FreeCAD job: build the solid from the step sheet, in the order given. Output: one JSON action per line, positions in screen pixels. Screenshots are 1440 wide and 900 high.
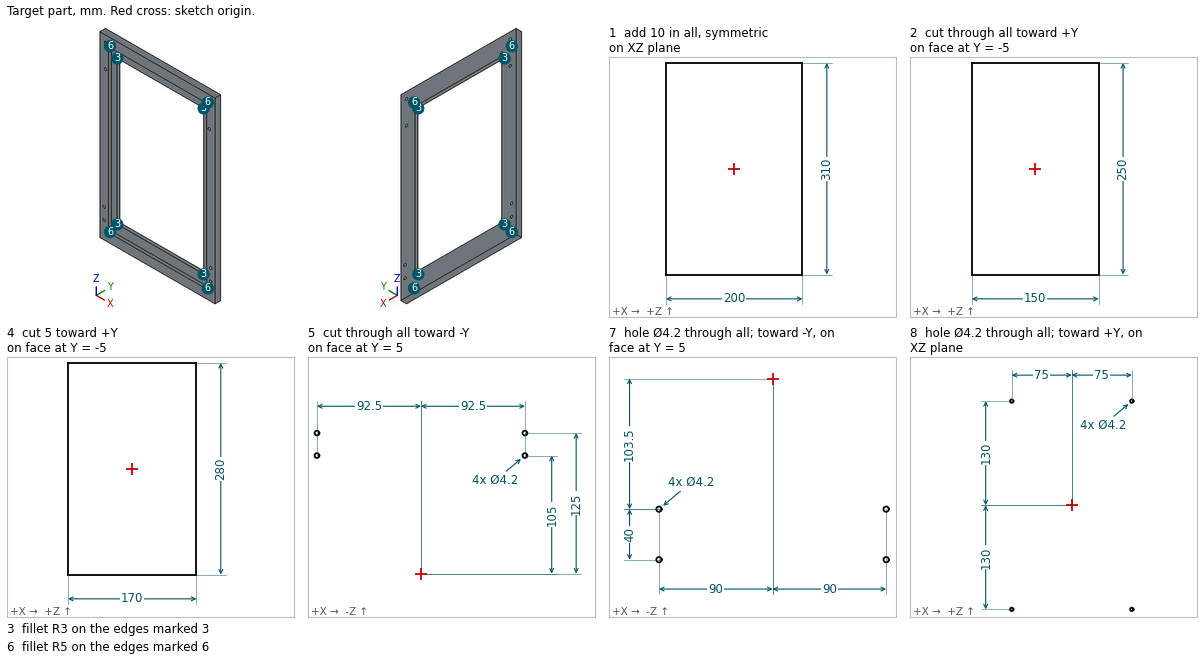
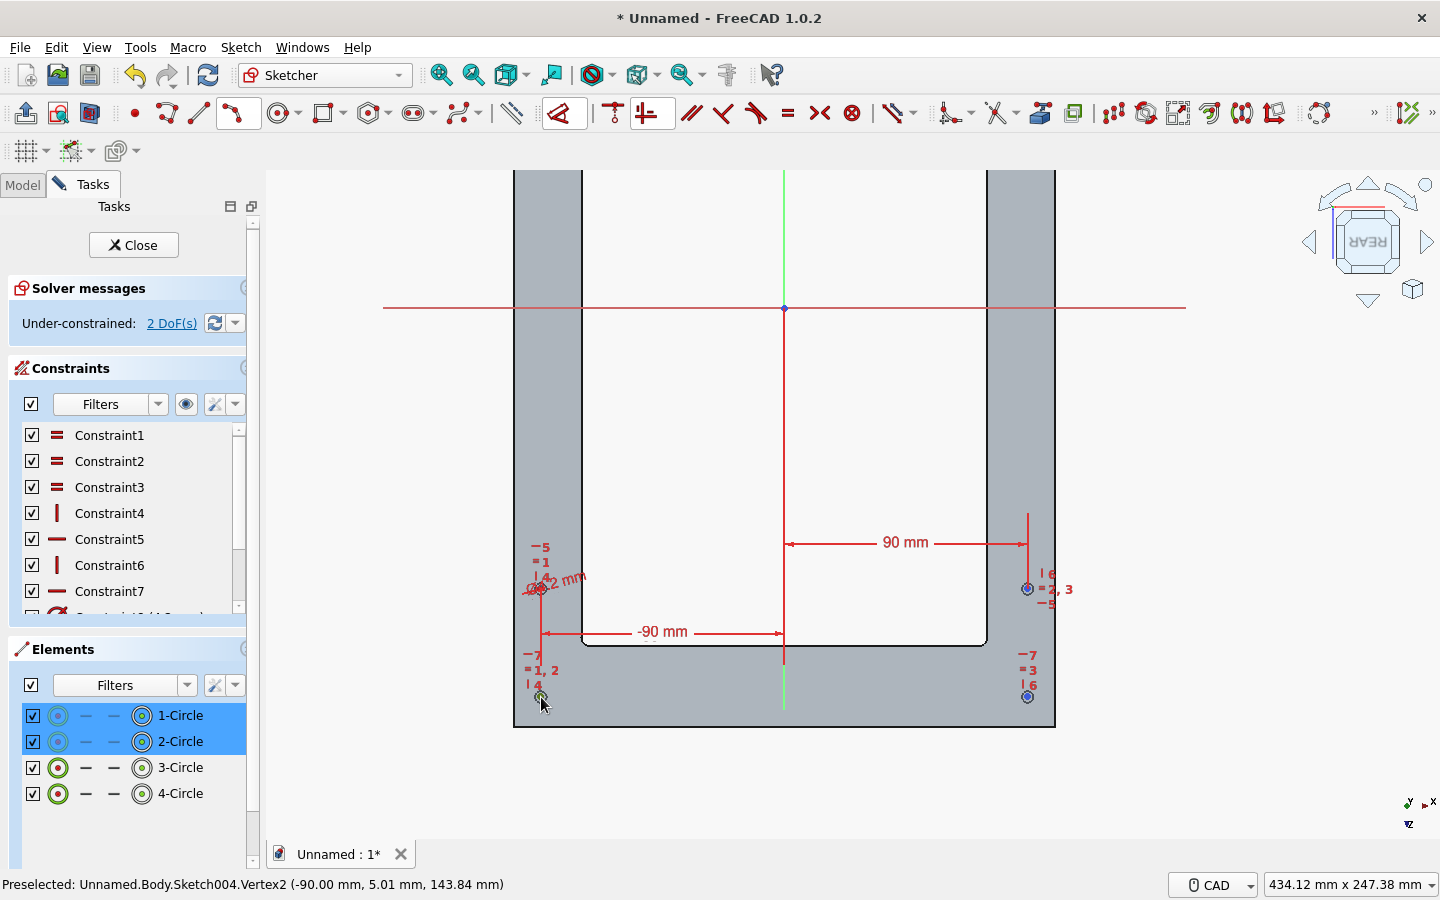
{"action": "key", "text": "i"}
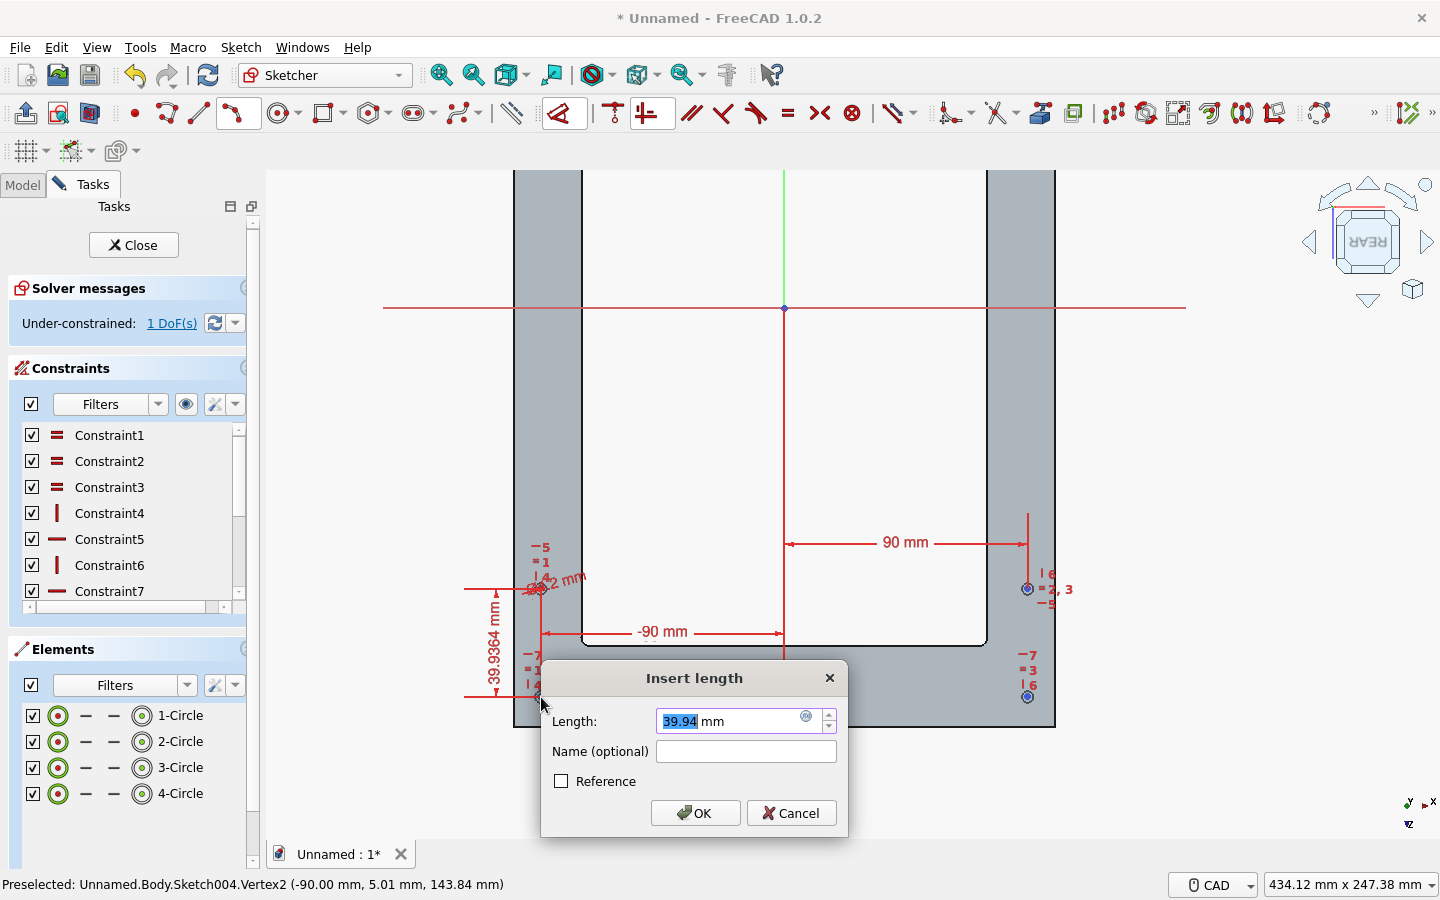
{"action": "type", "text": "40"}
{"action": "key", "text": "Return"}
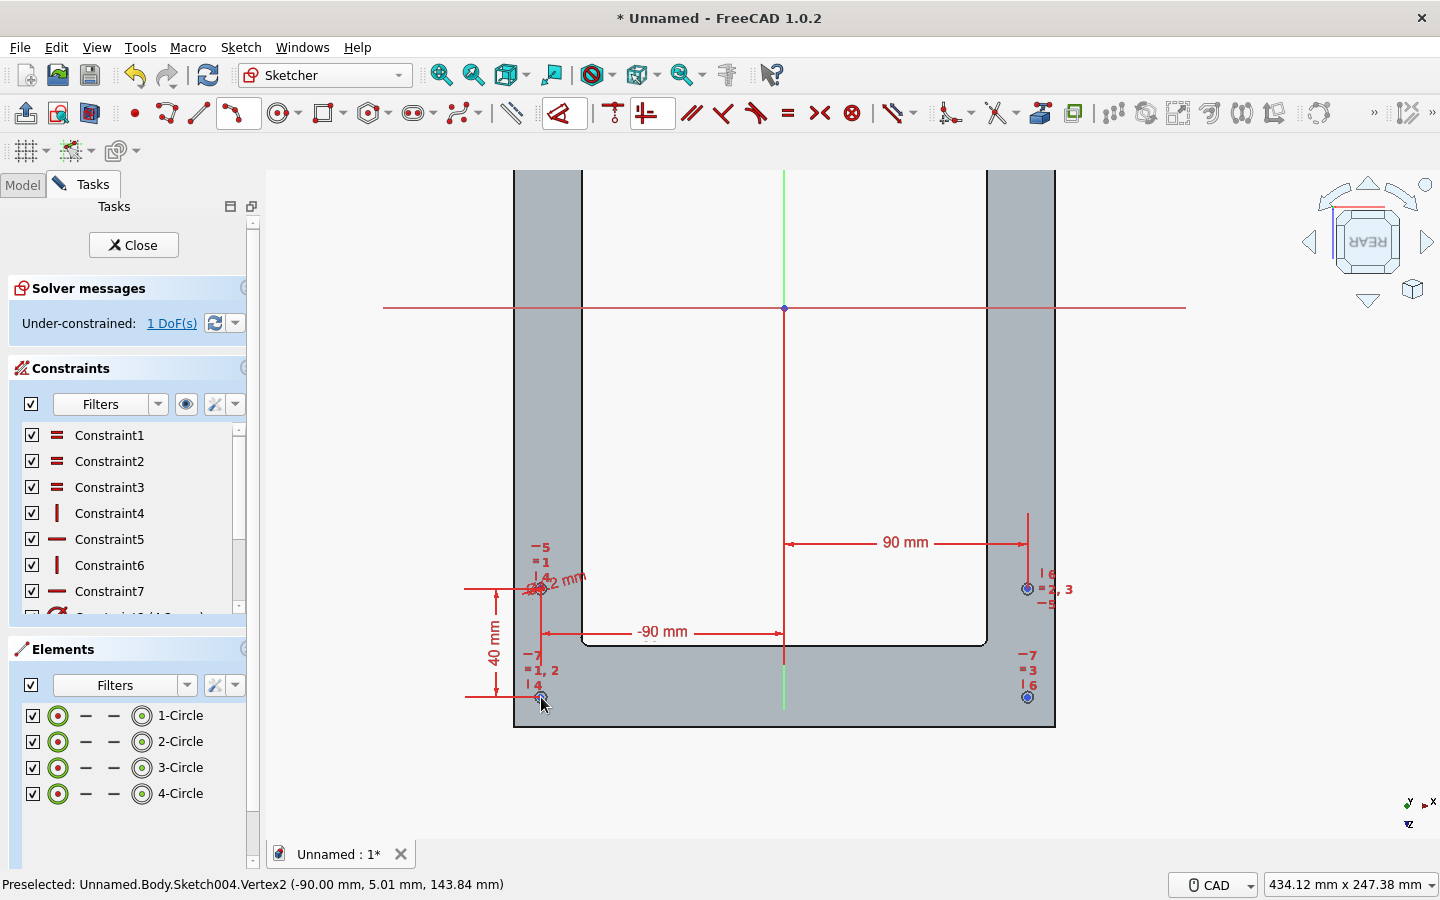
{"action": "left_click", "coordinate": [541, 589]}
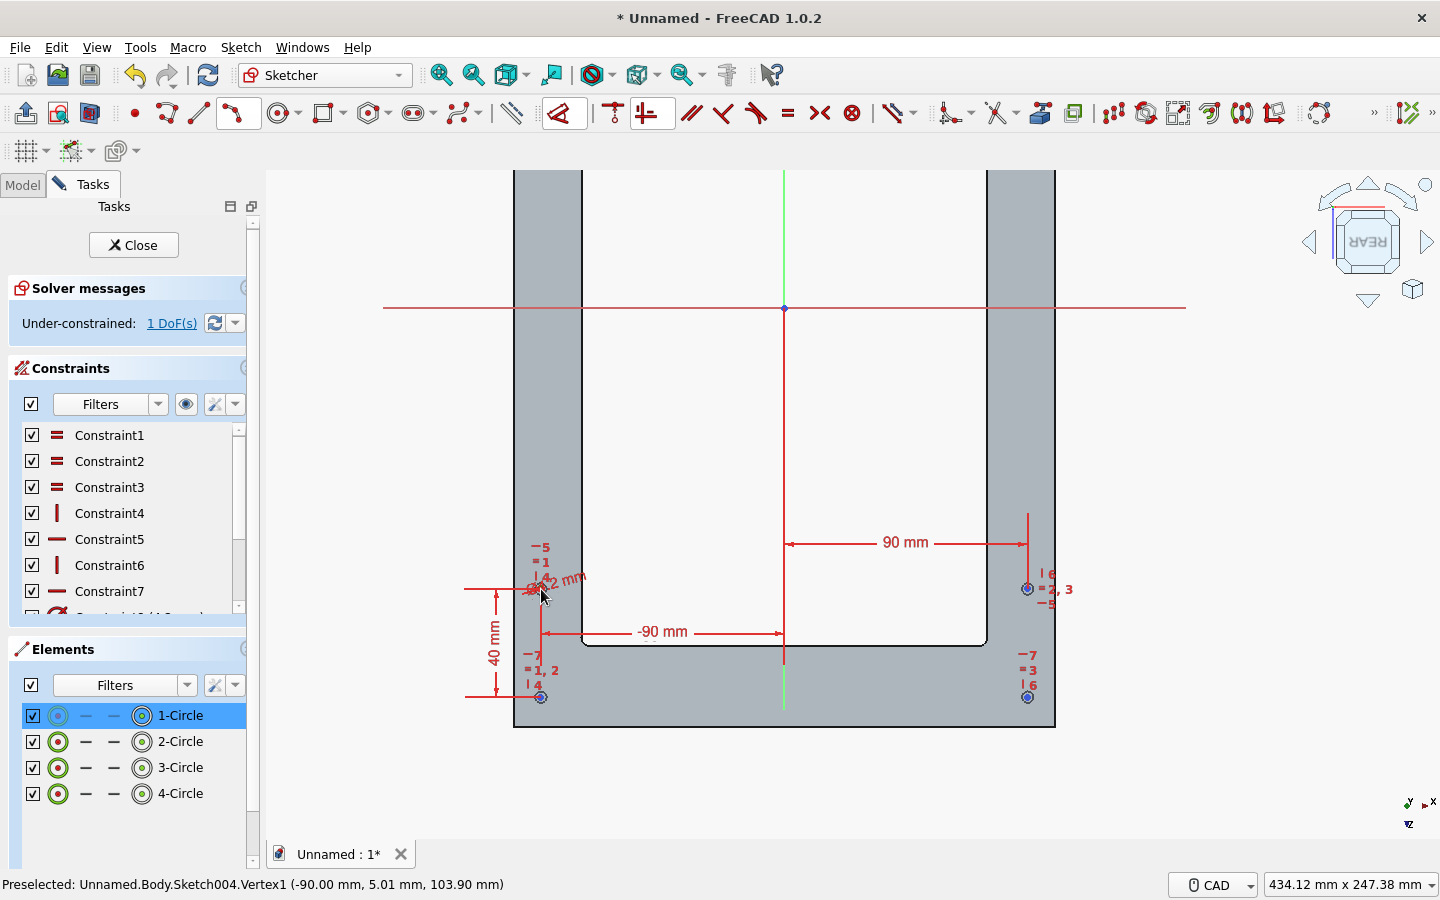
{"action": "key", "text": "i"}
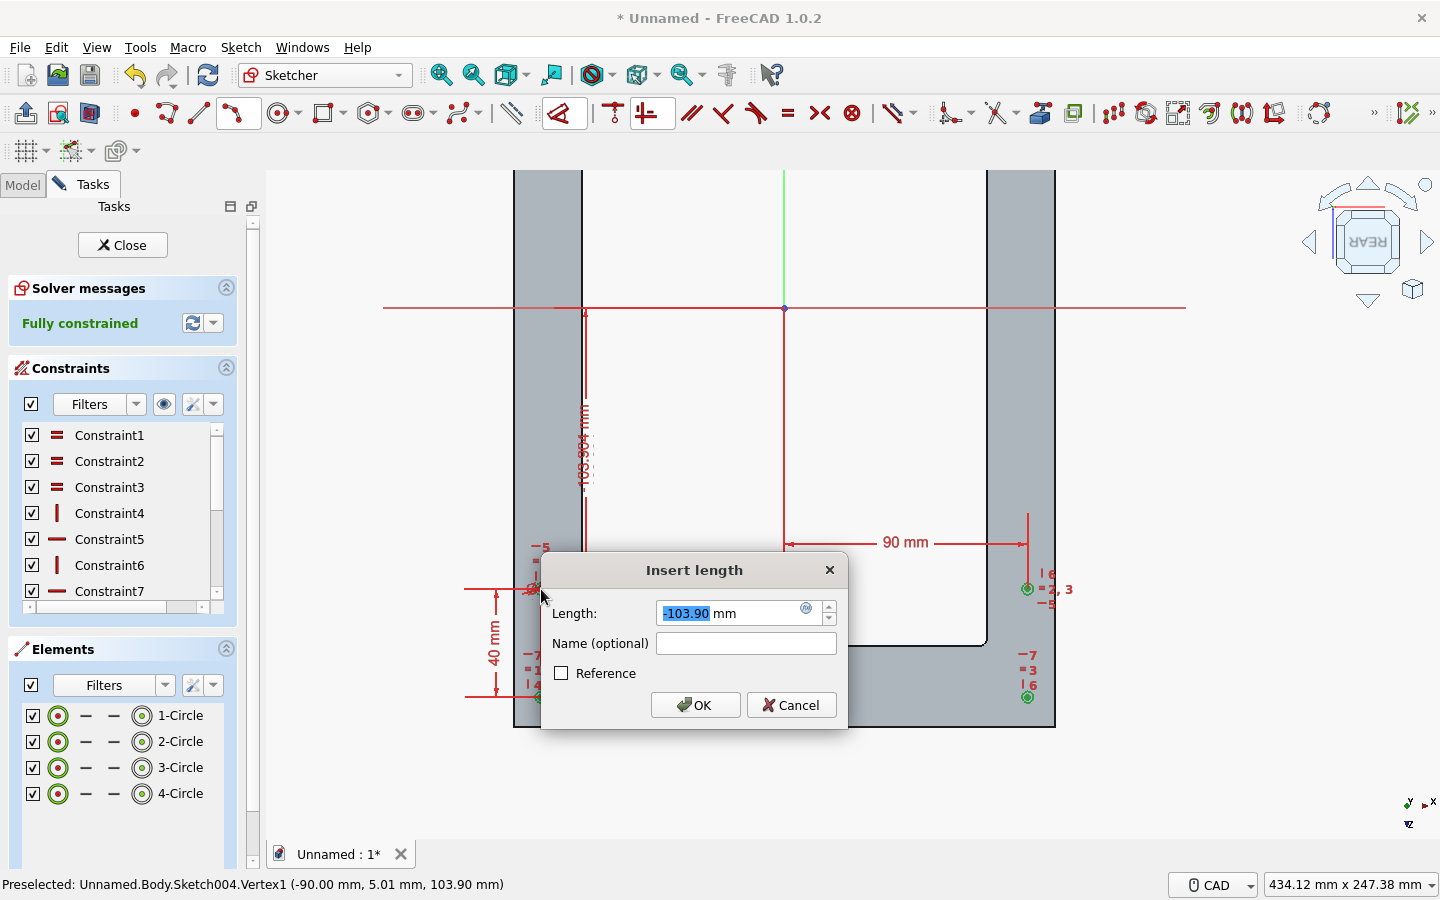
{"action": "type", "text": "-103.5"}
{"action": "key", "text": "Return"}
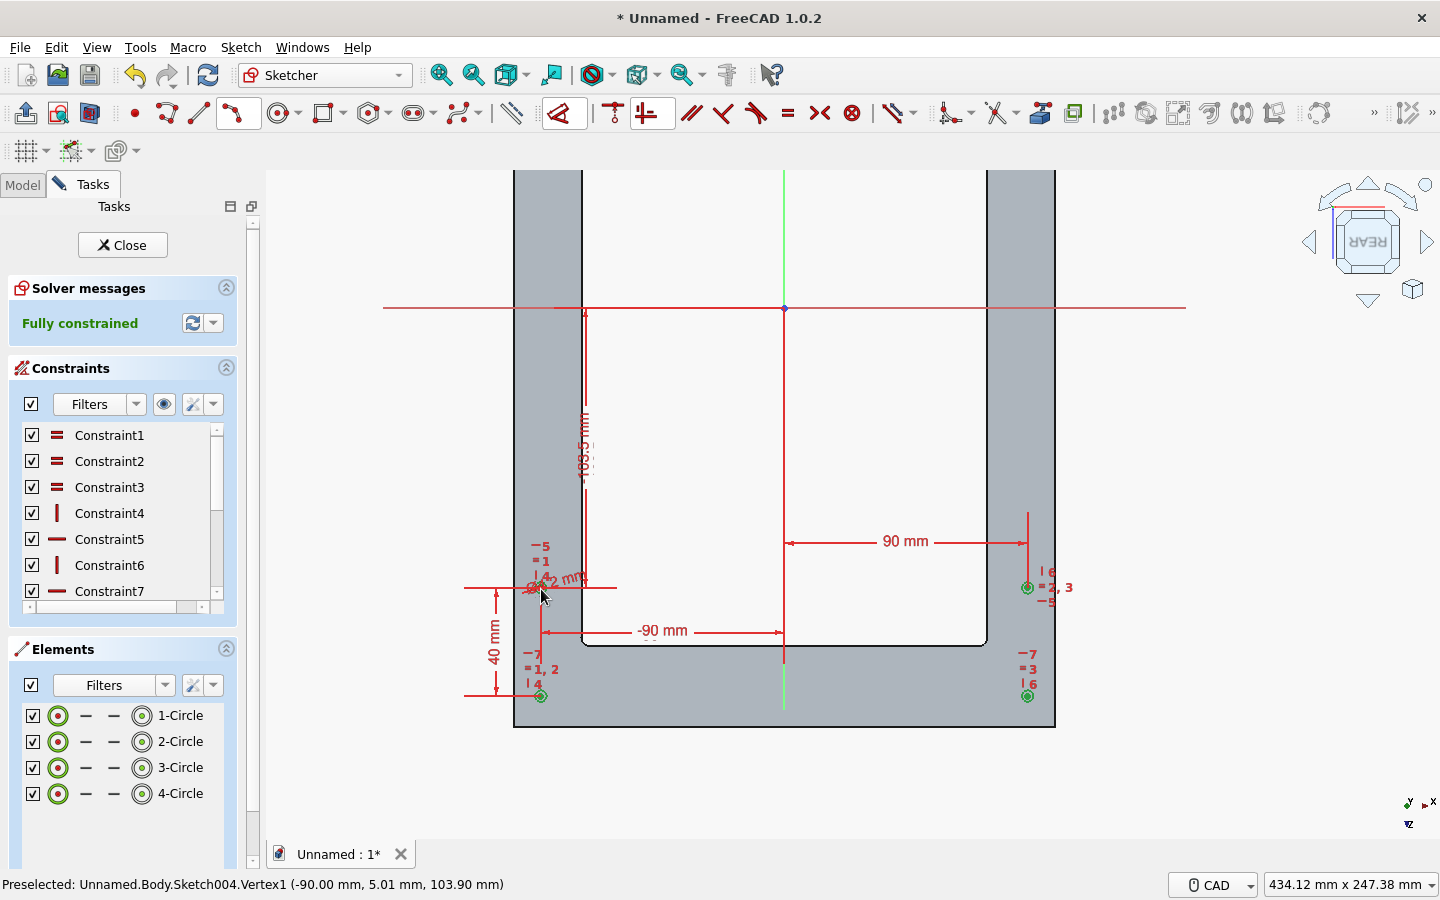
{"action": "left_click", "coordinate": [123, 245]}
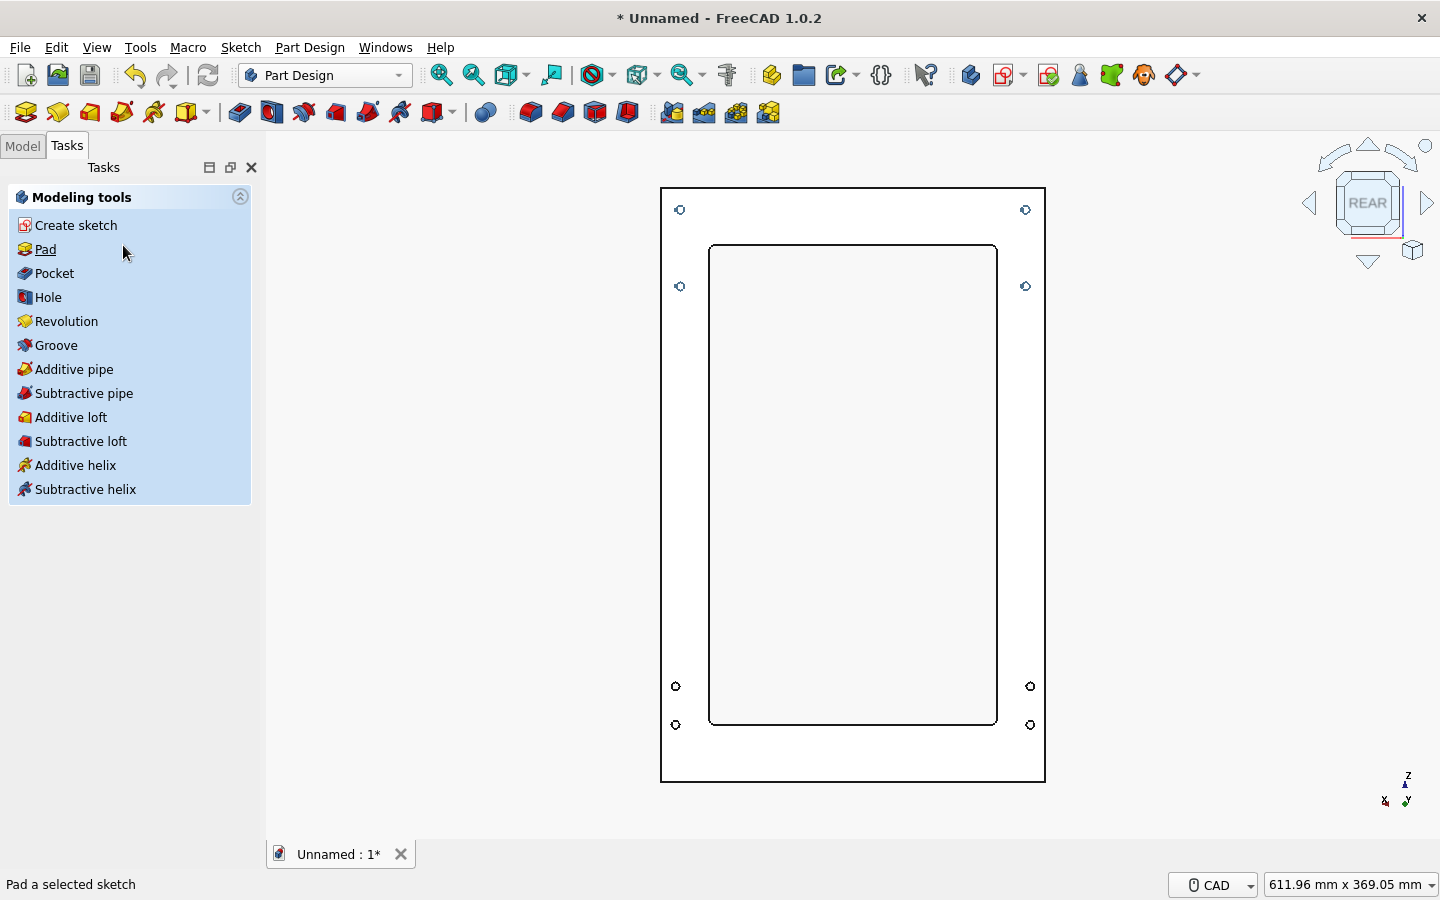
{"action": "left_click", "coordinate": [272, 112]}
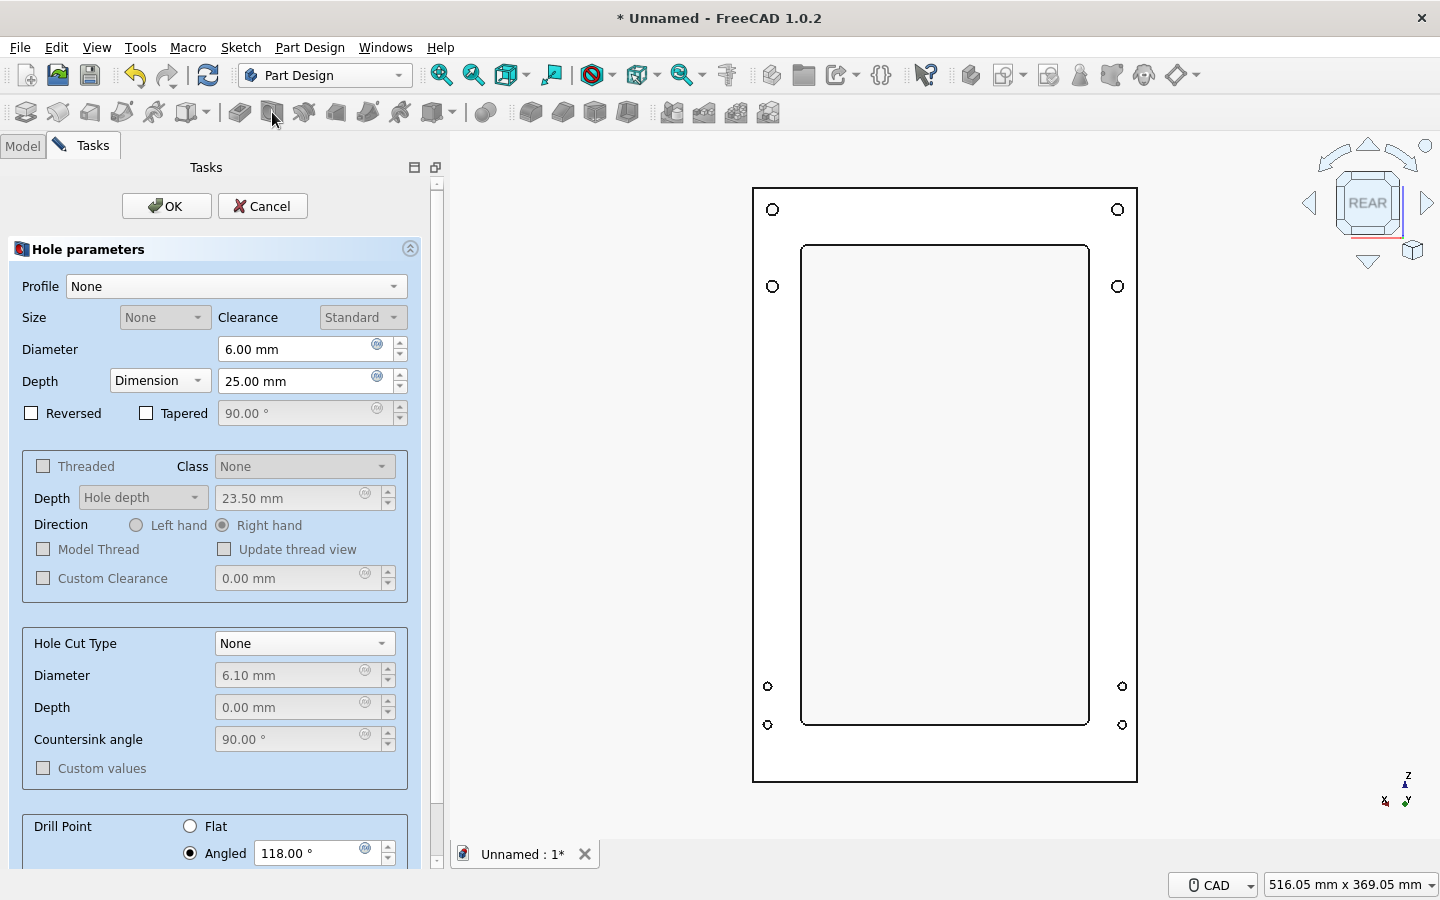
{"action": "triple_click", "coordinate": [305, 349]}